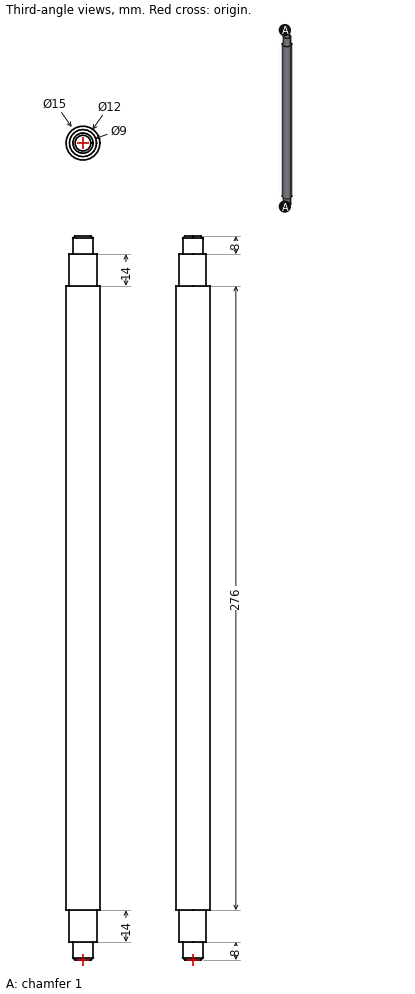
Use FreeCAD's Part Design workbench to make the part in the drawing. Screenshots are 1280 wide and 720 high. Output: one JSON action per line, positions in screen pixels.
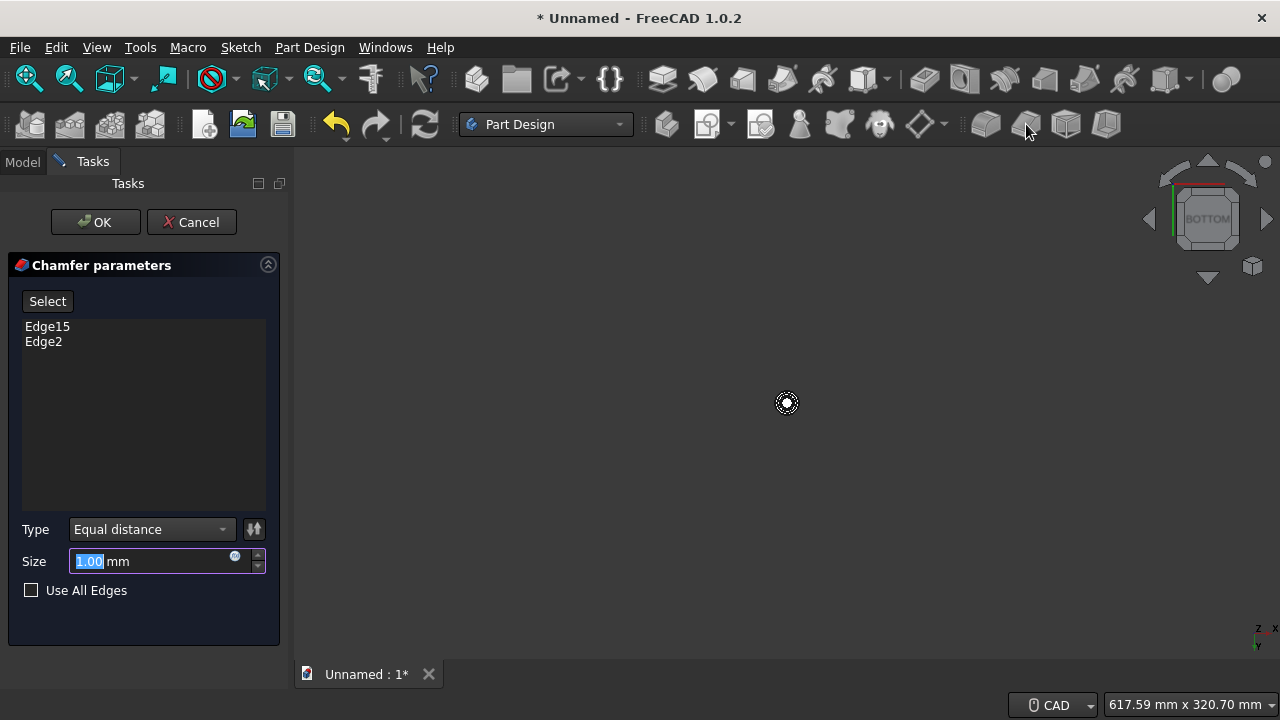
{"action": "type", "text": "1"}
{"action": "key", "text": "Tab"}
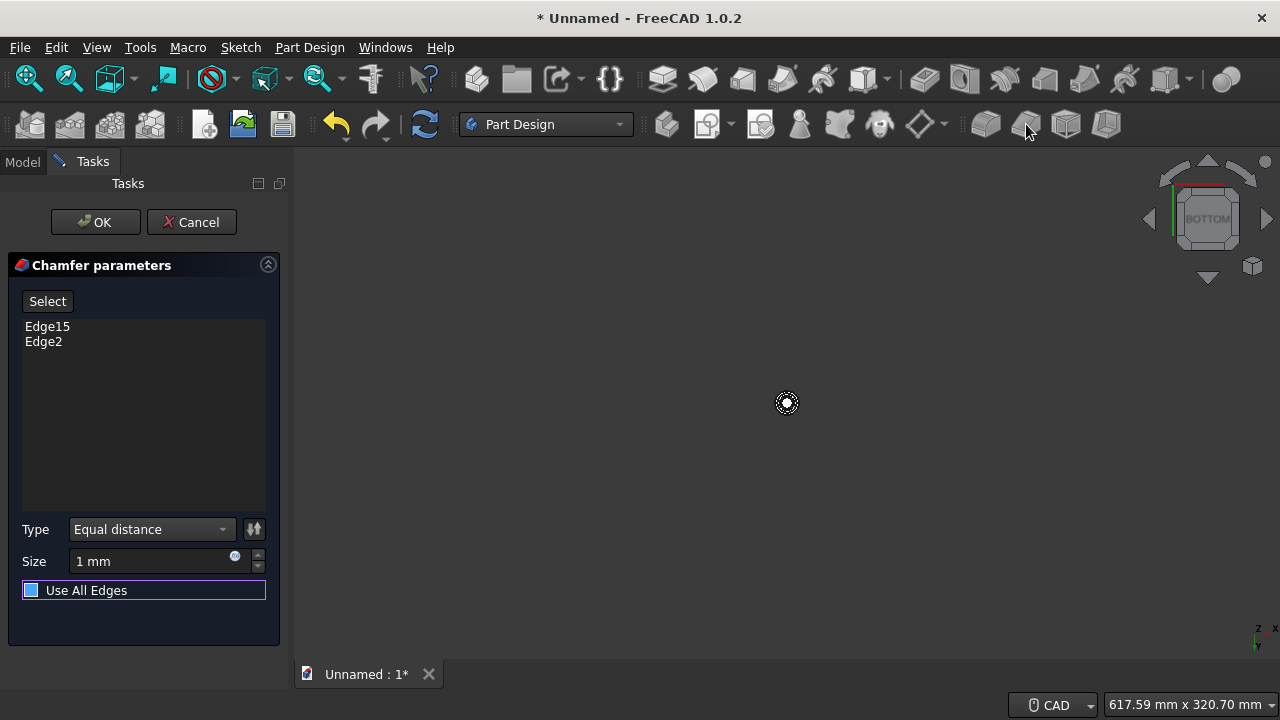
{"action": "left_click", "coordinate": [96, 222]}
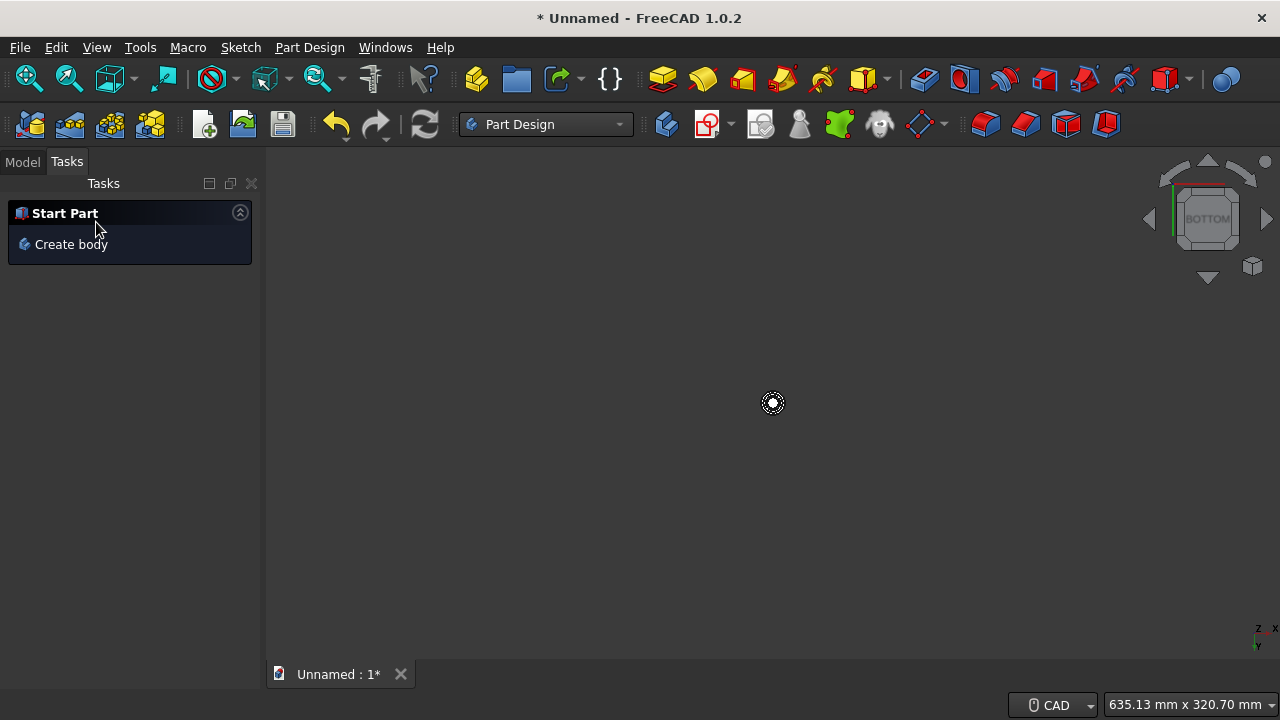
{"action": "key", "text": "0"}